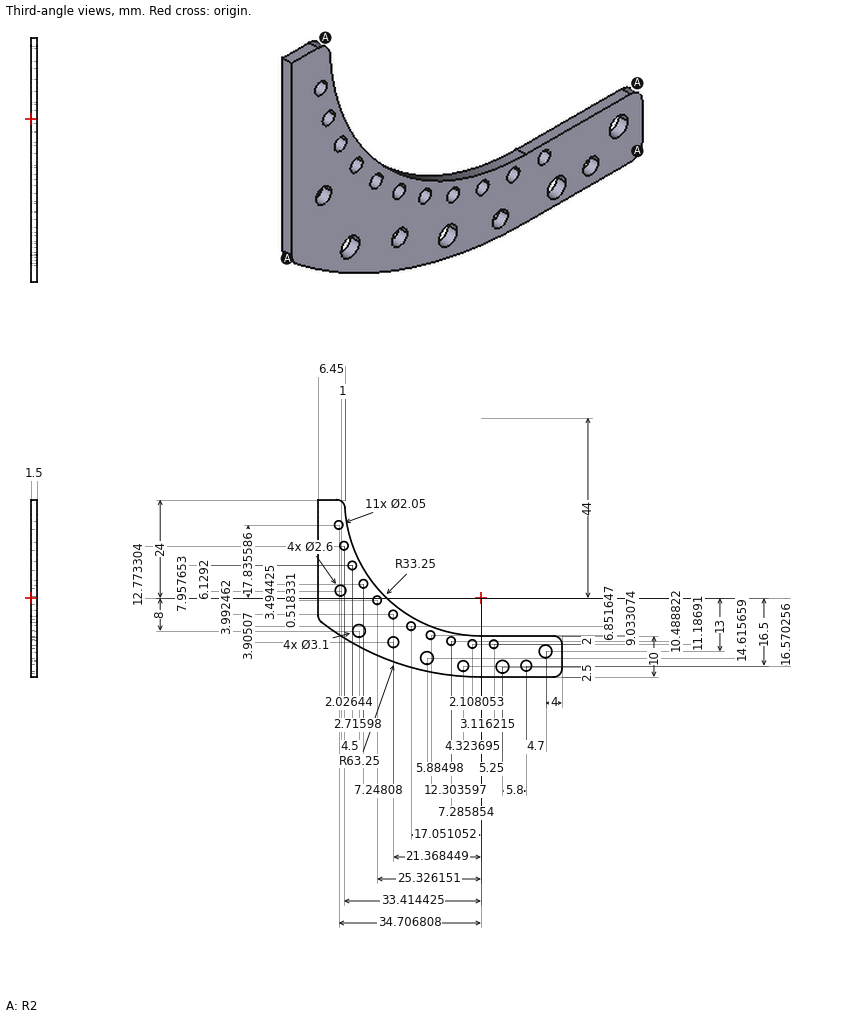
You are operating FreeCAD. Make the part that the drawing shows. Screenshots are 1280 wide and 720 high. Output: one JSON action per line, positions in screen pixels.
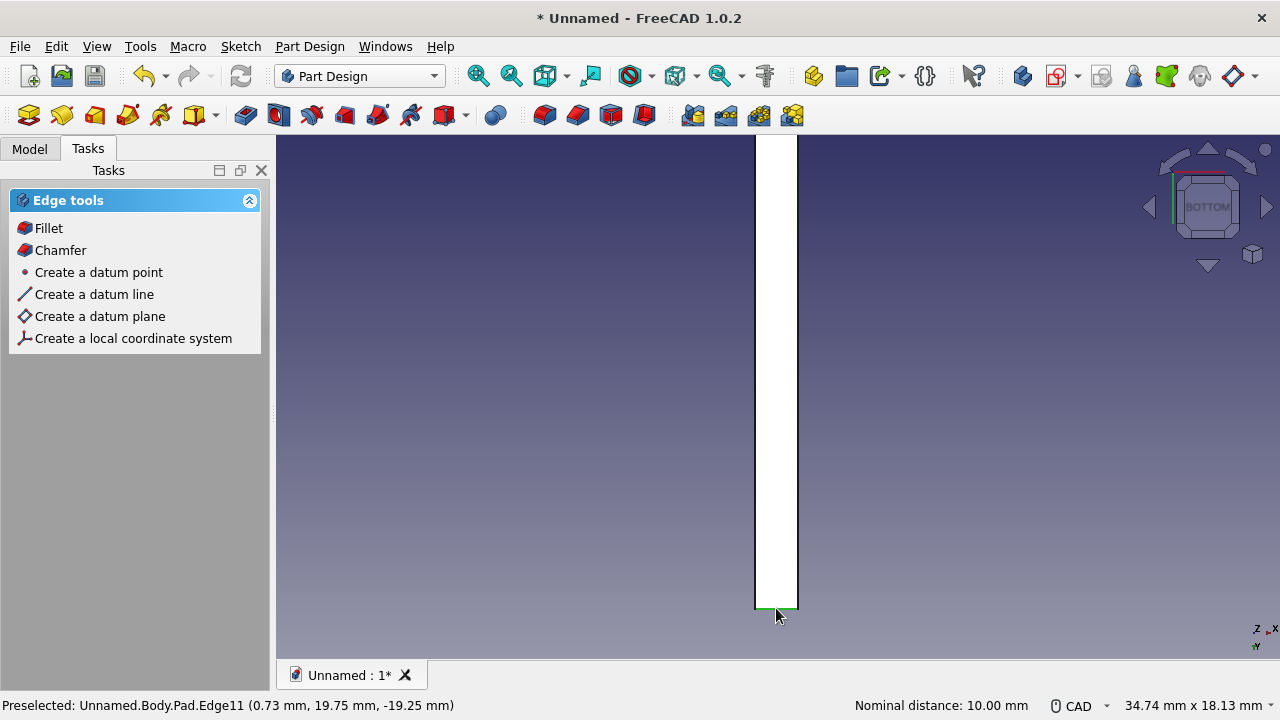
{"action": "left_click", "coordinate": [479, 76]}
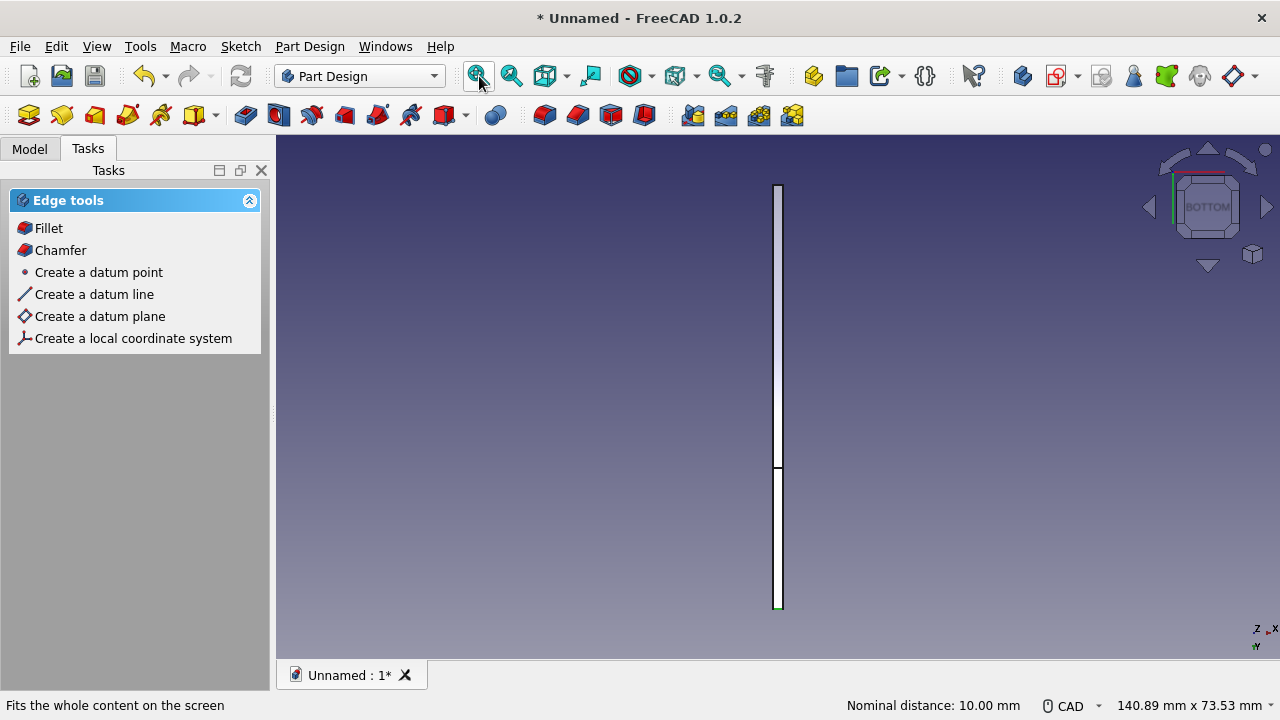
{"action": "key", "text": "4"}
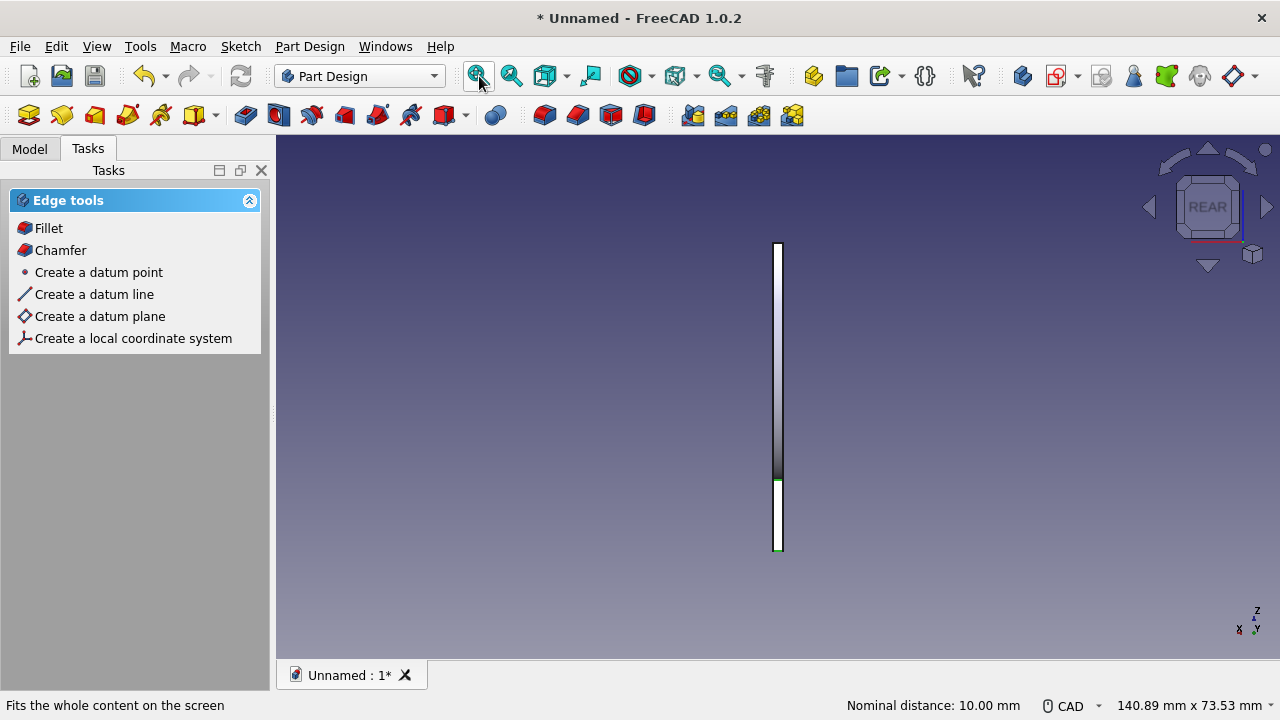
{"action": "scroll", "coordinate": [778, 450], "scroll_direction": "up", "scroll_amount": 7}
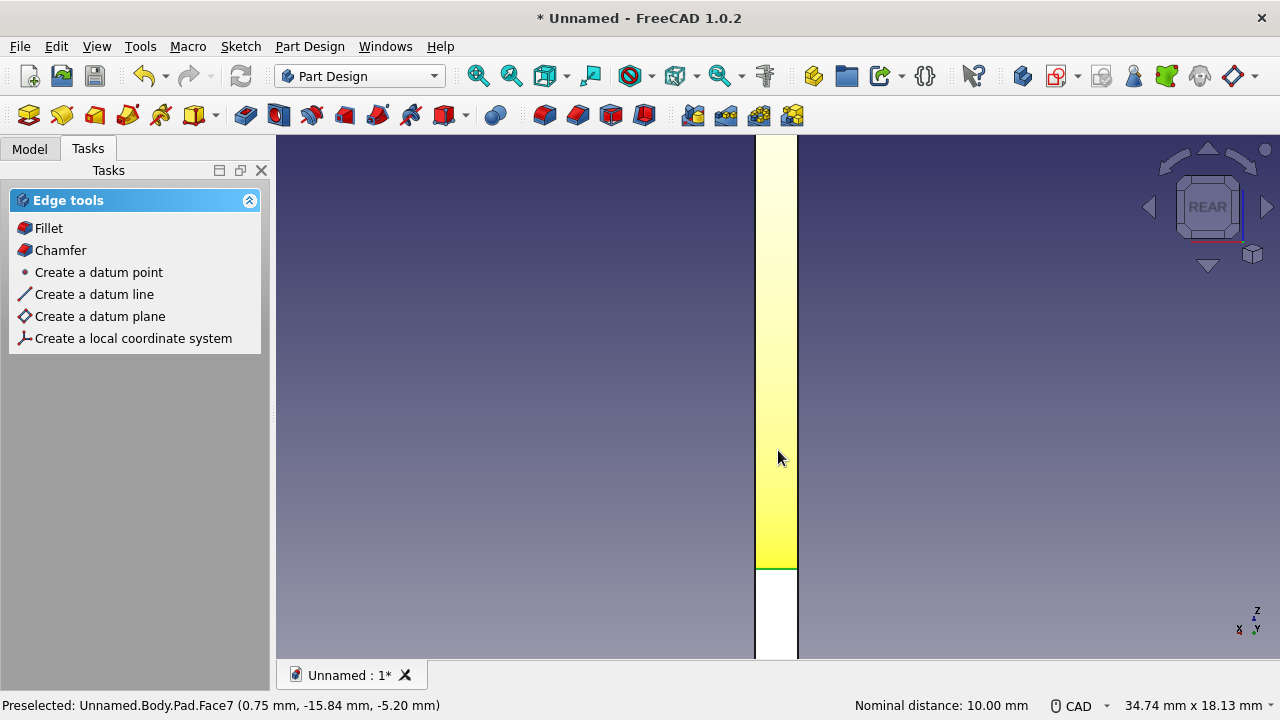
{"action": "left_click", "coordinate": [479, 76]}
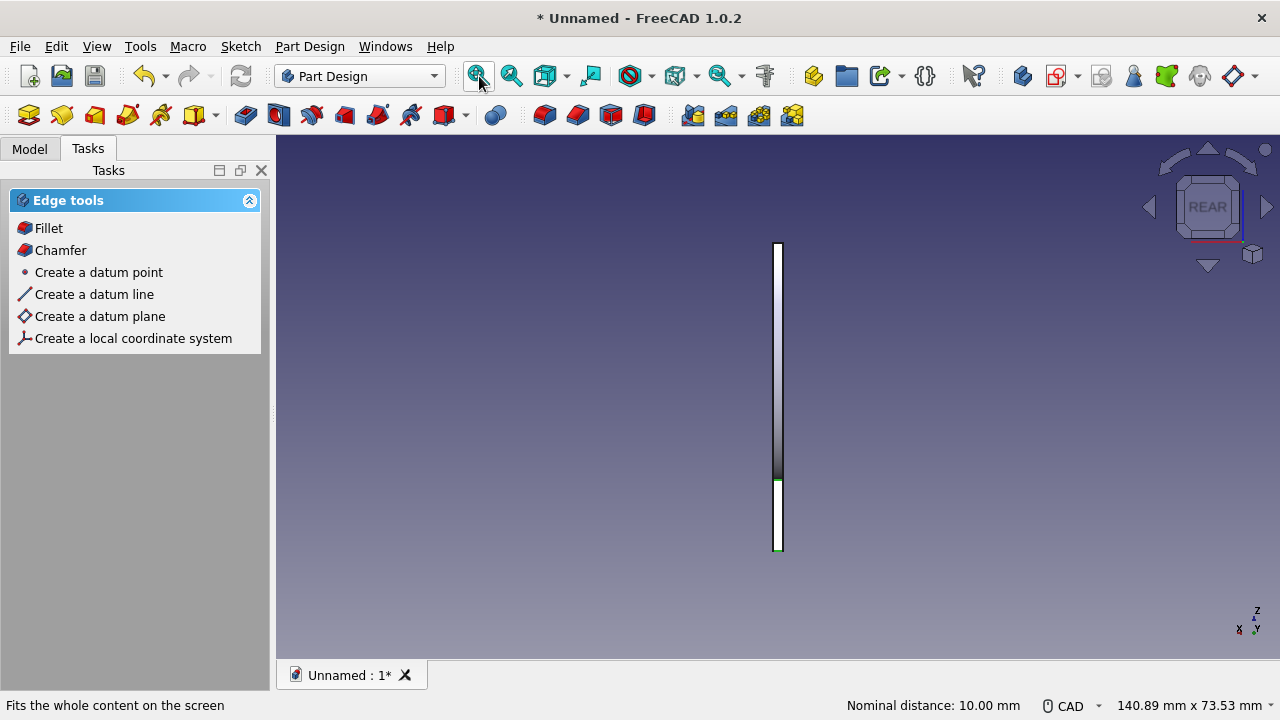
{"action": "key", "text": "6"}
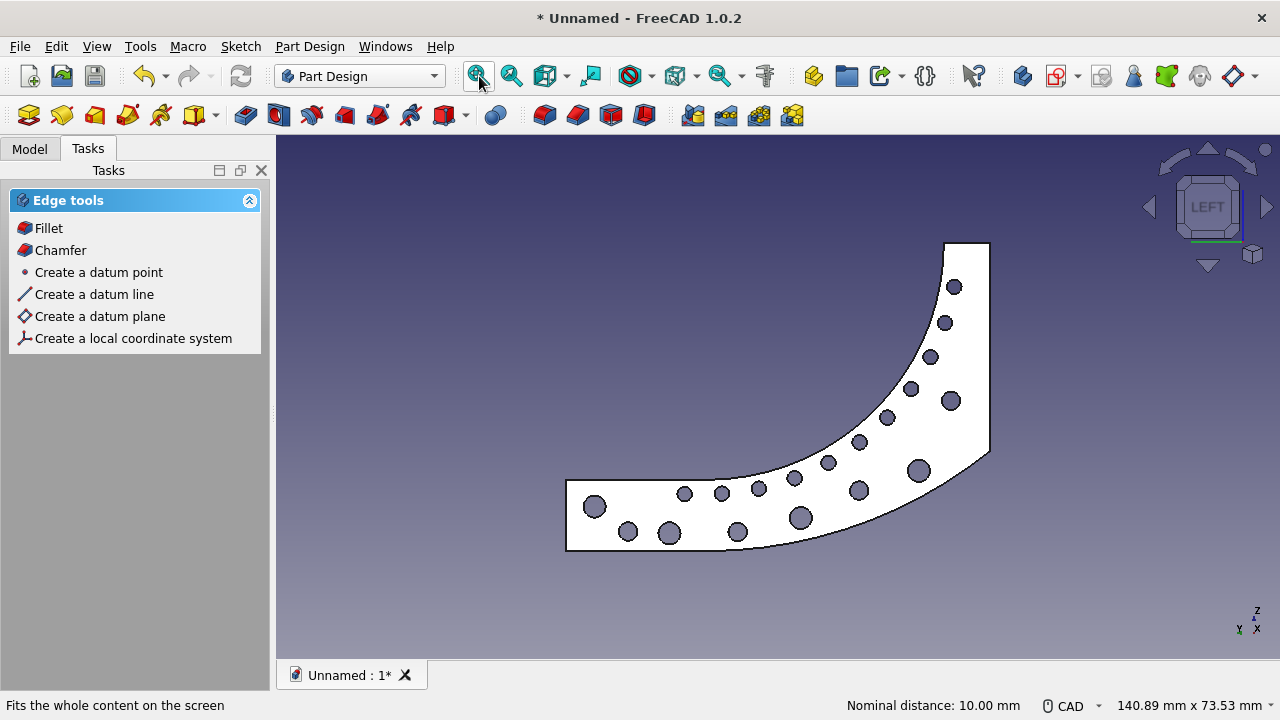
{"action": "scroll", "coordinate": [990, 450], "scroll_direction": "up", "scroll_amount": 7}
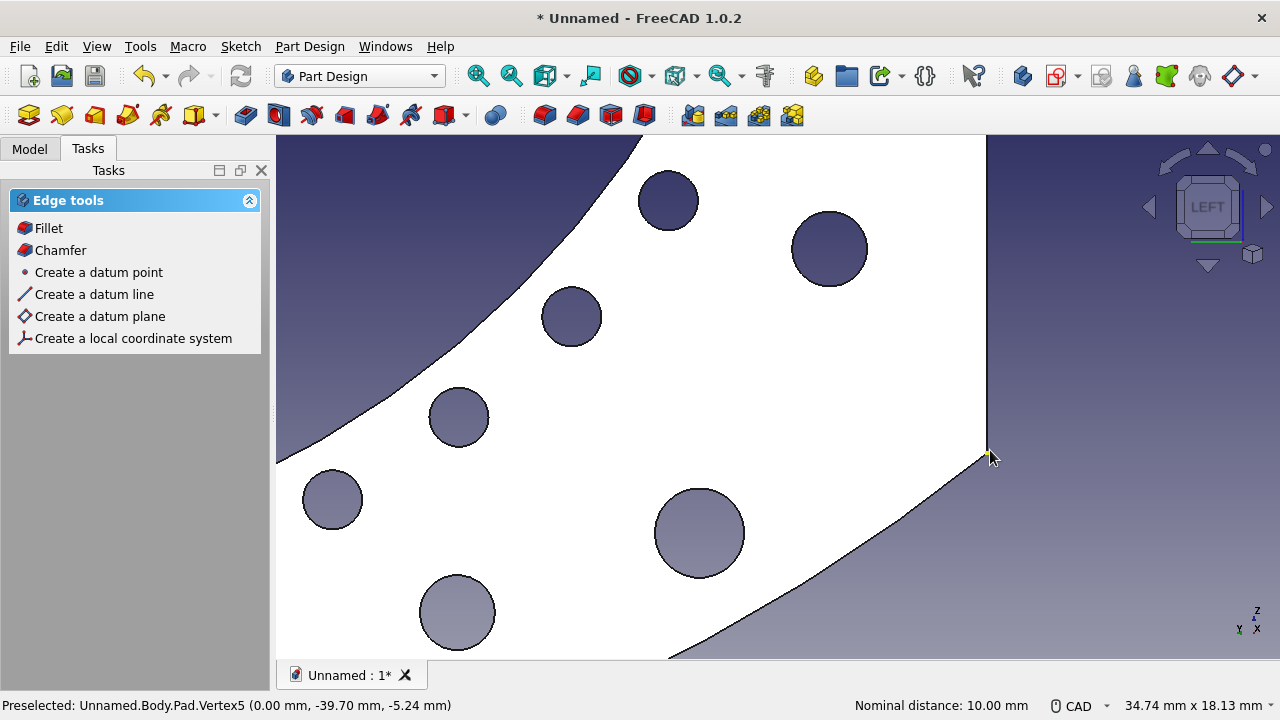
{"action": "left_click", "coordinate": [479, 76]}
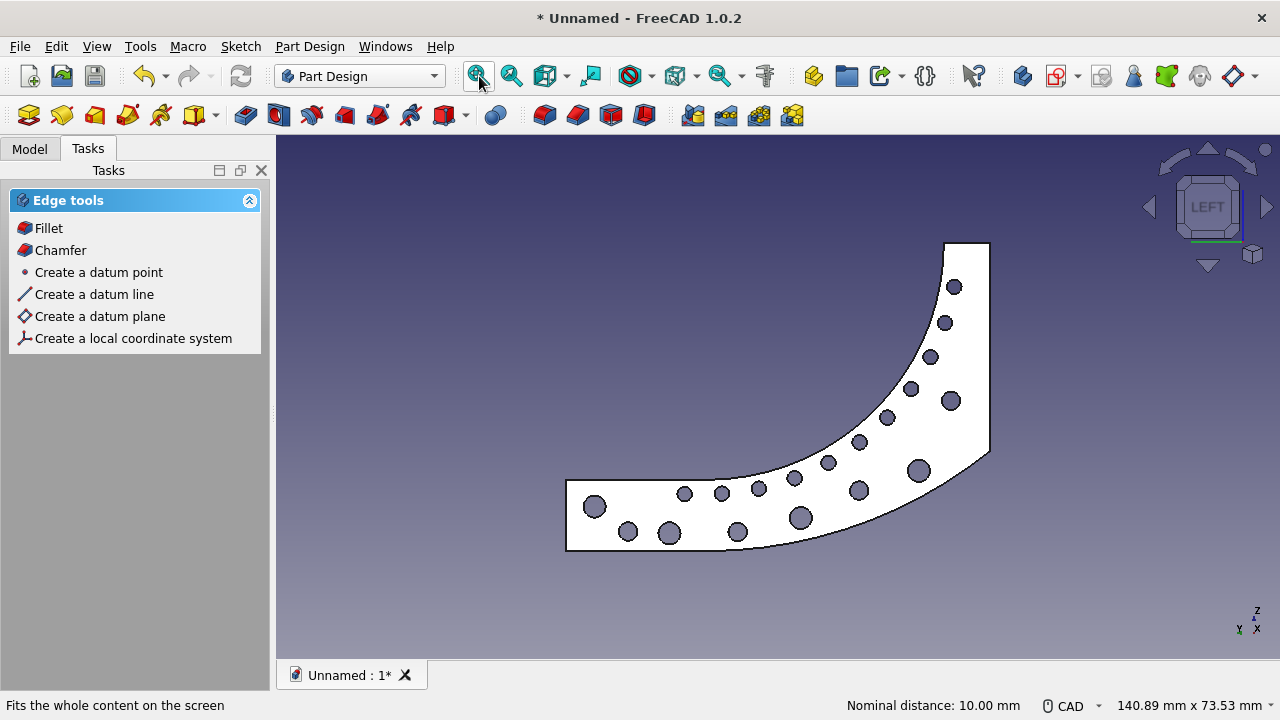
{"action": "key", "text": "v 3"}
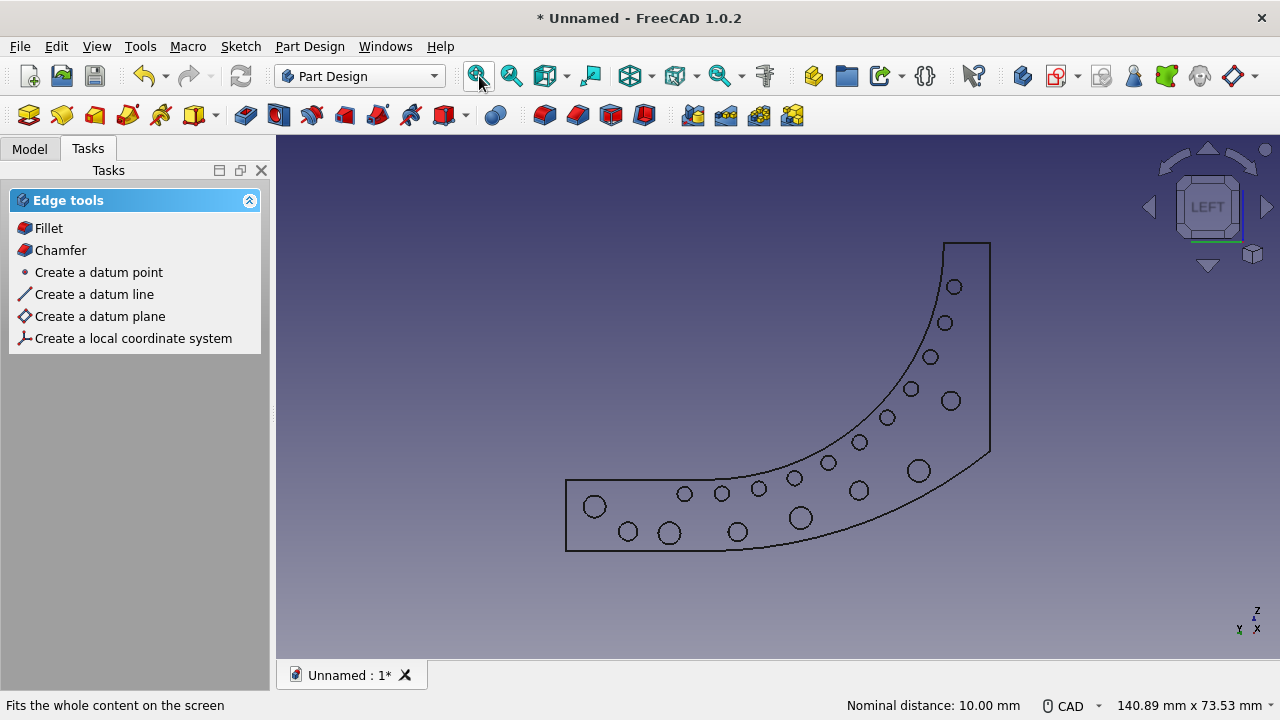
{"action": "key", "text": "0"}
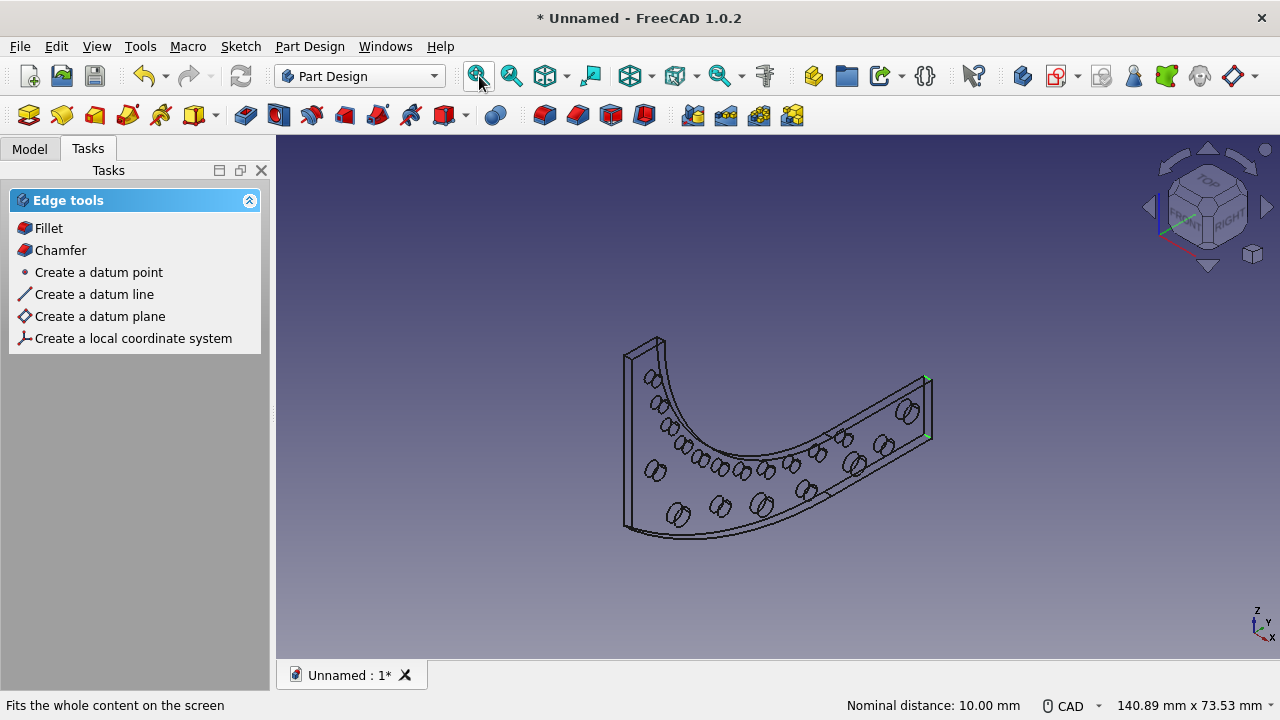
{"action": "scroll", "coordinate": [628, 527], "scroll_direction": "up", "scroll_amount": 7}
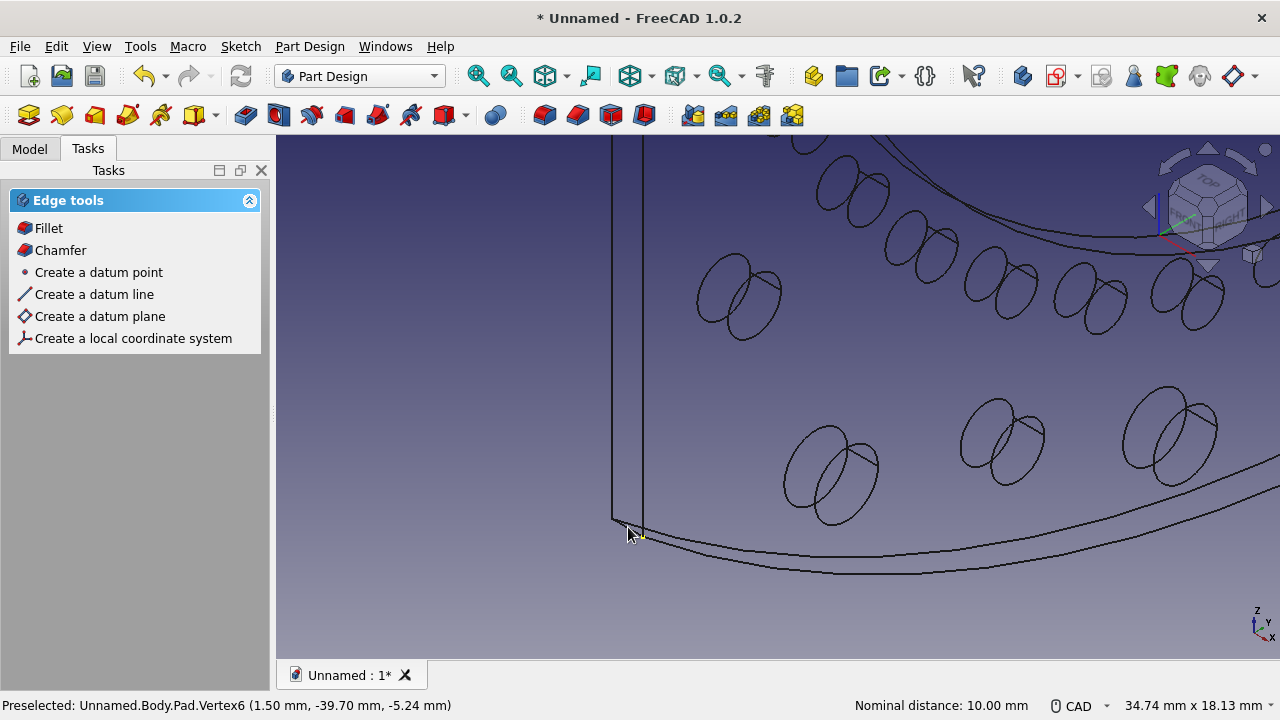
{"action": "left_click", "coordinate": [628, 527], "text": "ctrl"}